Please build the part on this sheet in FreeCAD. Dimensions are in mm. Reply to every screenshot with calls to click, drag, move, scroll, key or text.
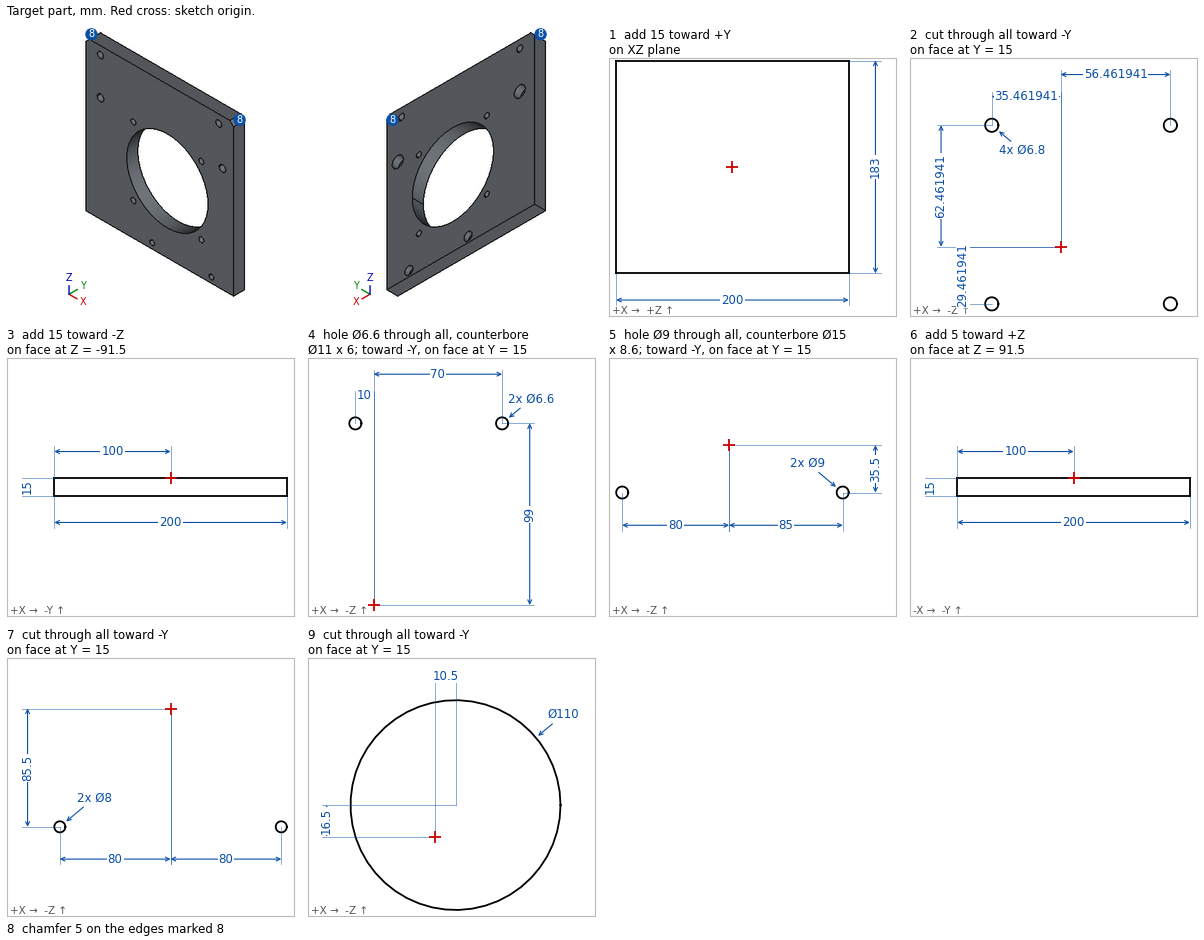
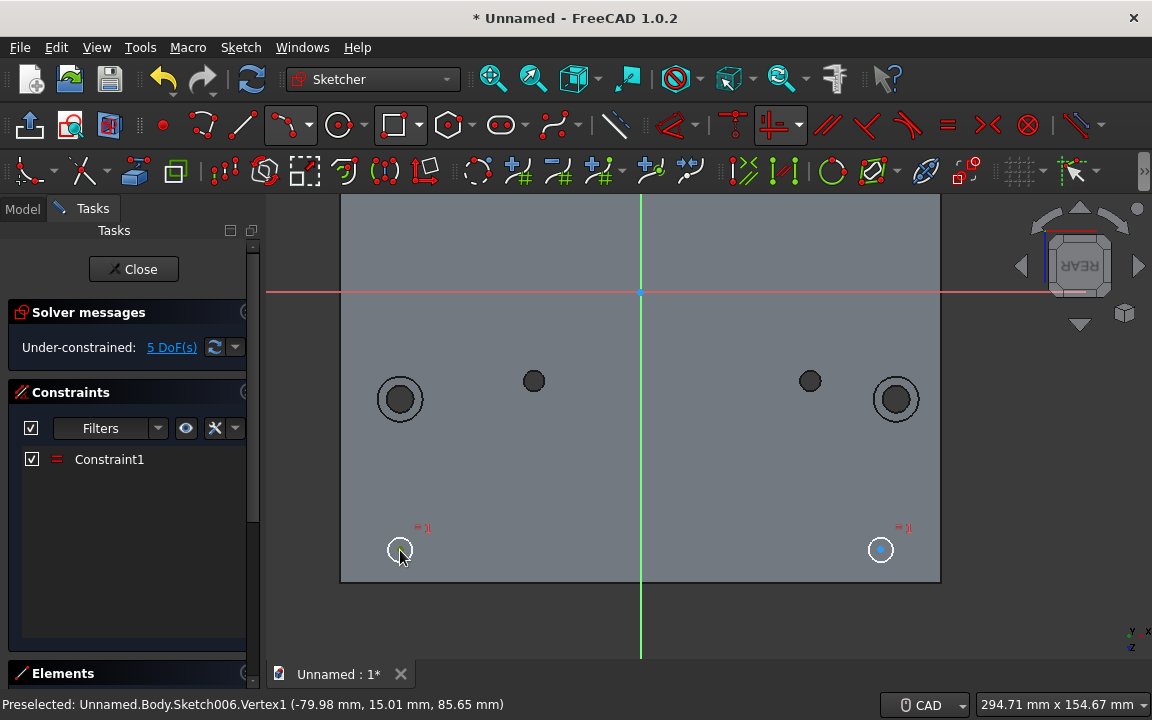
click(881, 550)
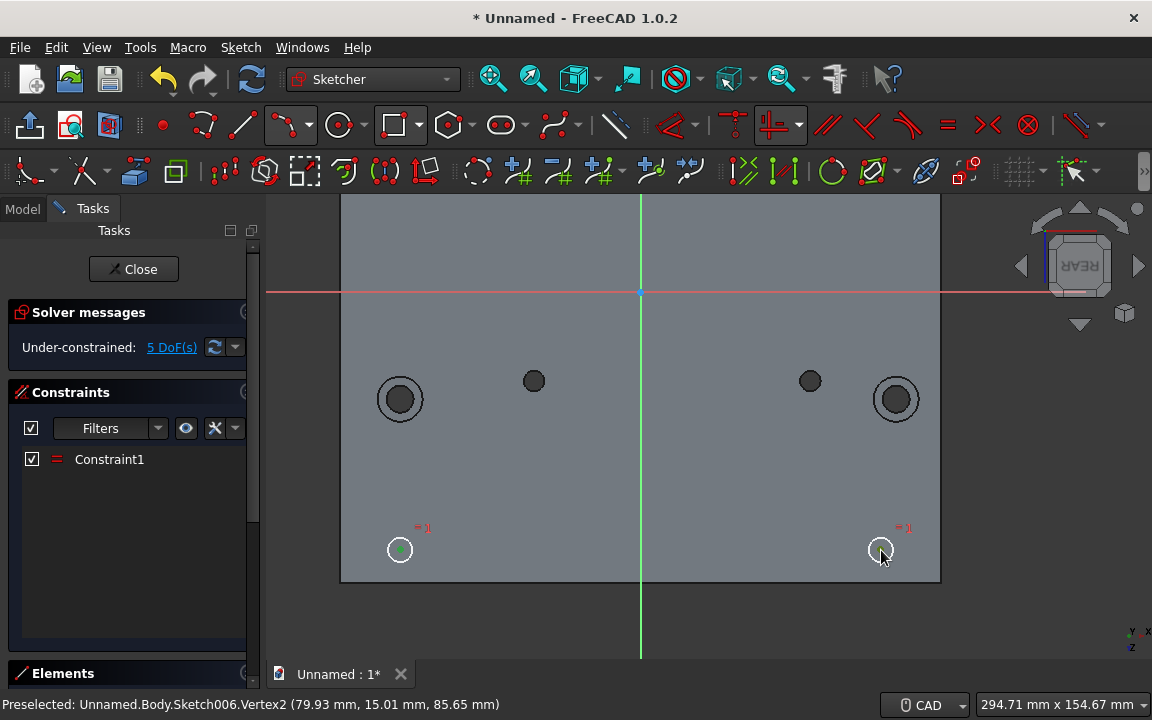
key(h)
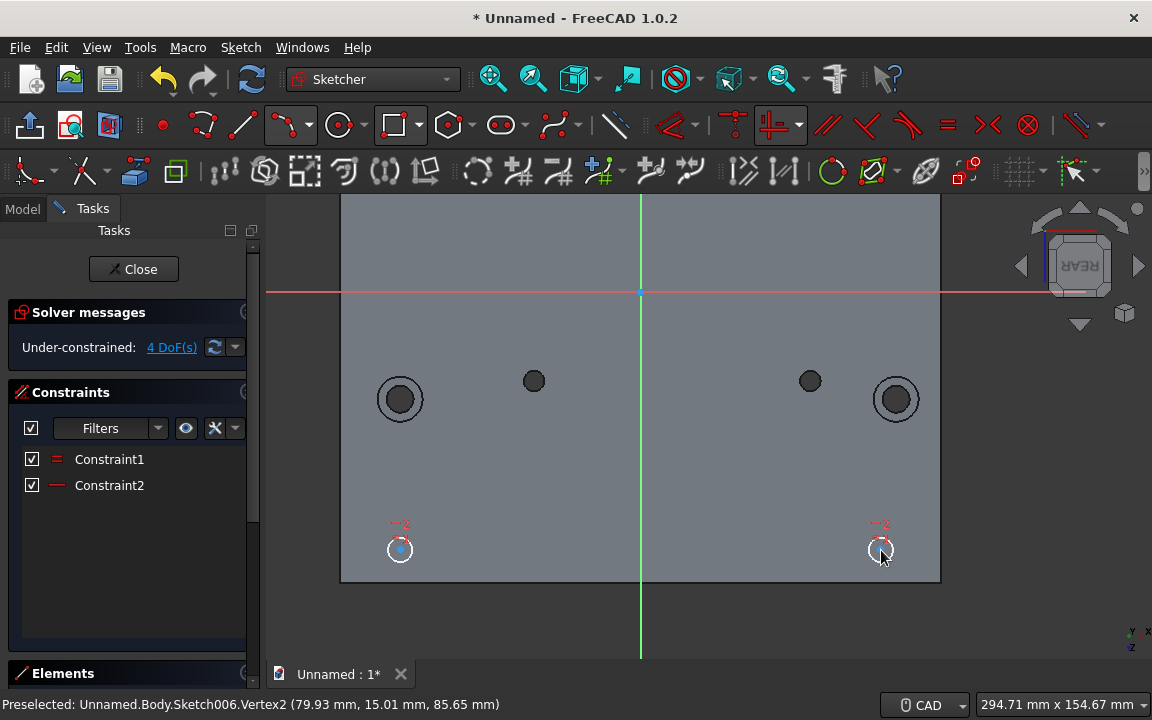
click(670, 126)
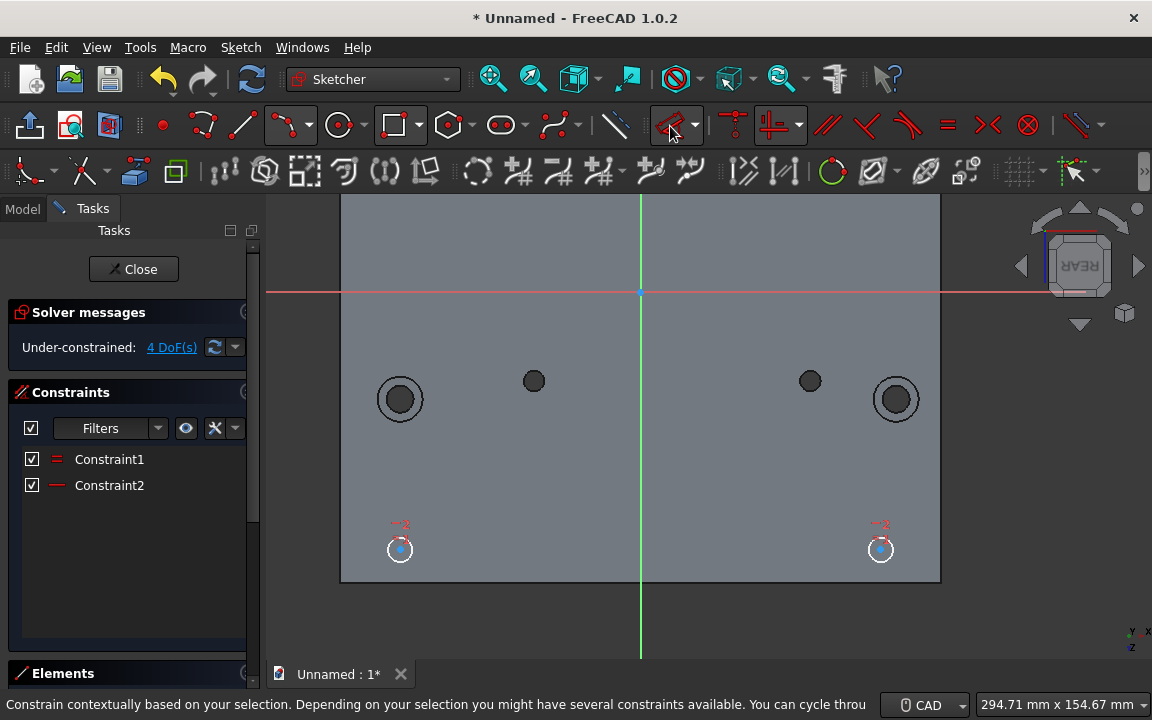
scroll(409, 541, up, 3)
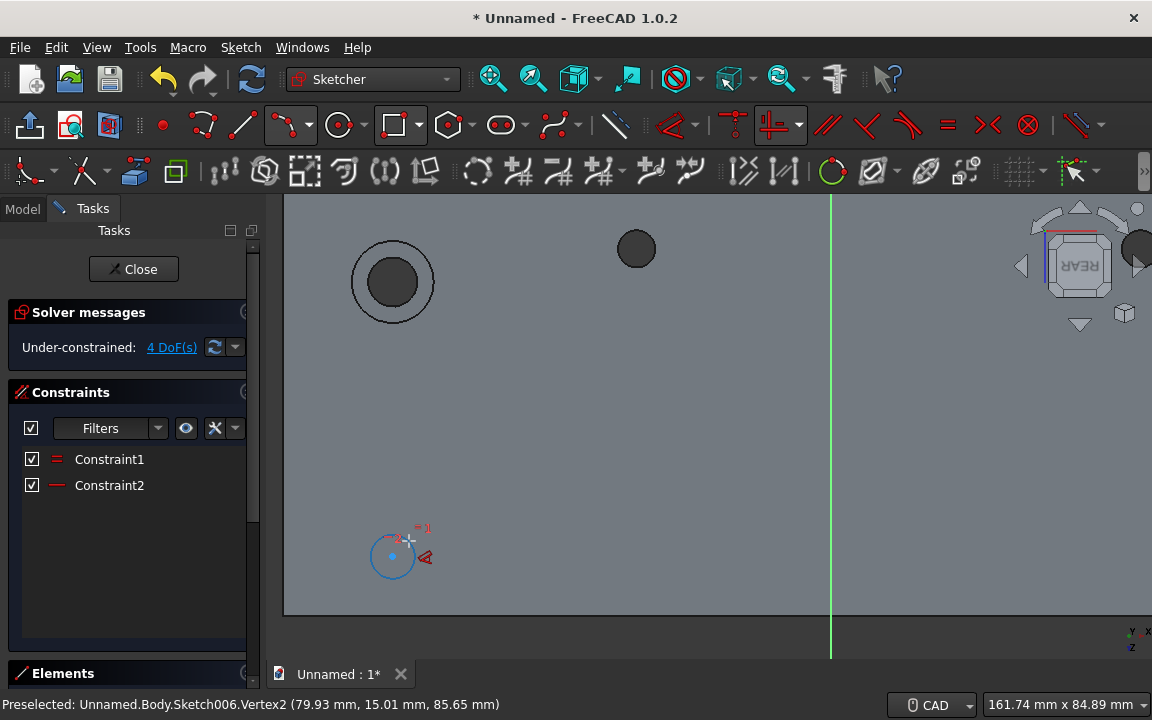
click(408, 541)
click(430, 518)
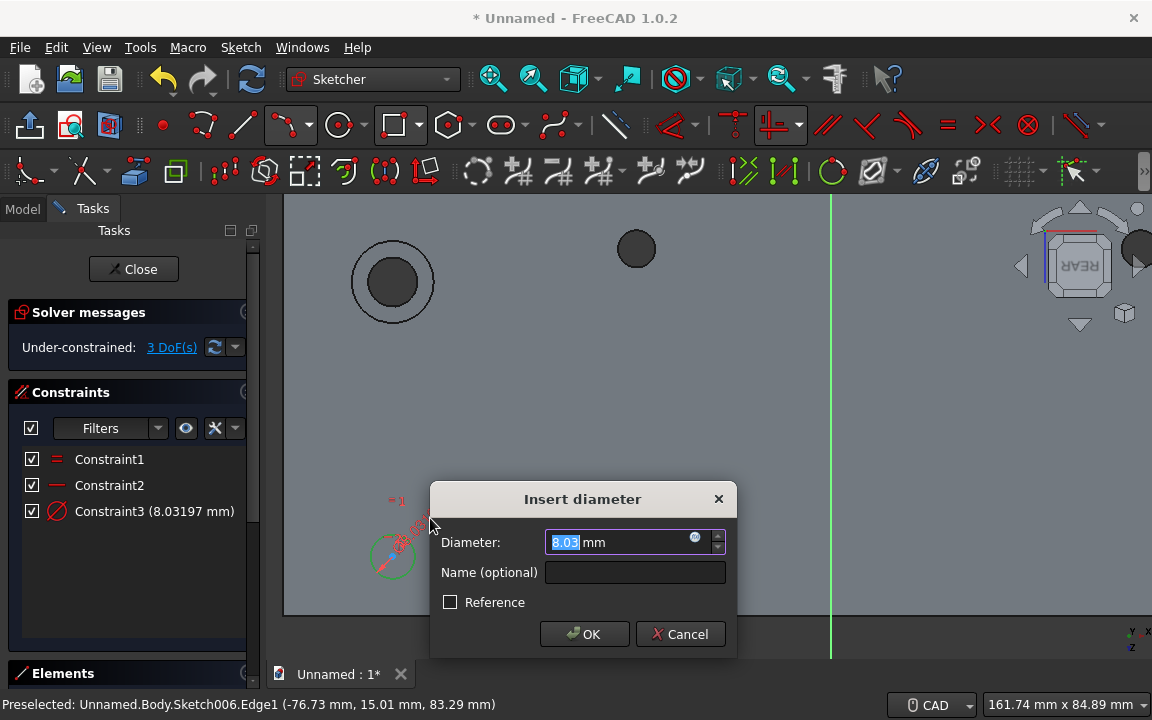
text(8)
key(Return)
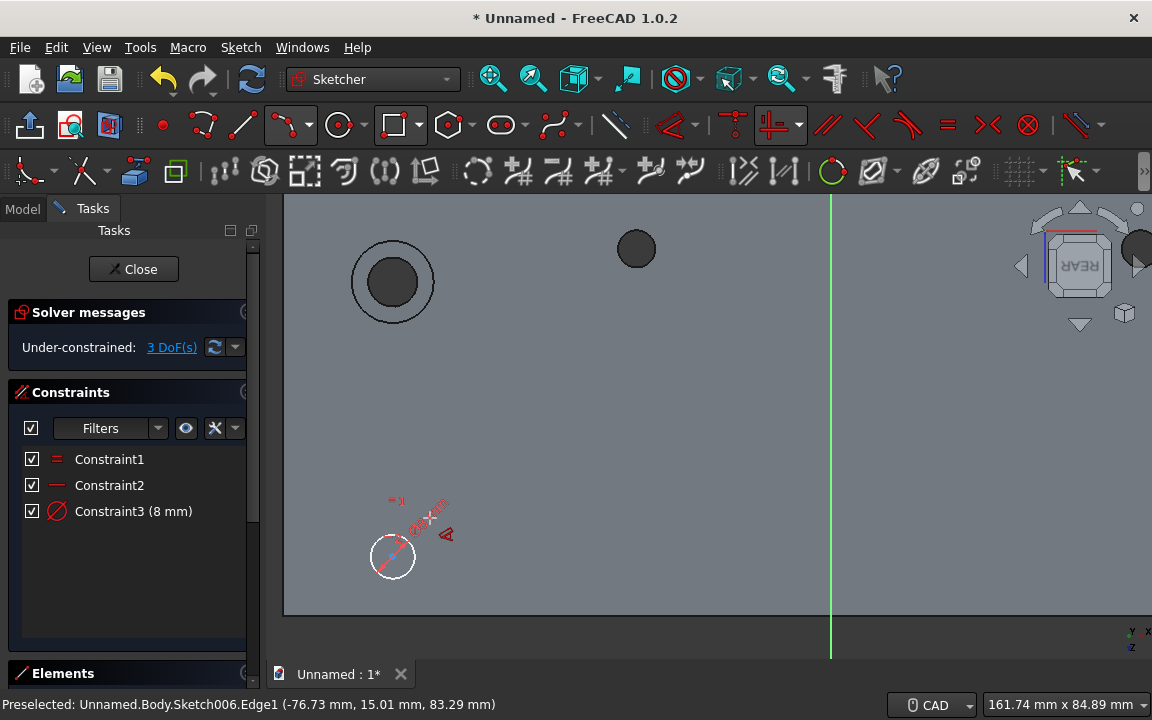
click(393, 557)
click(612, 591)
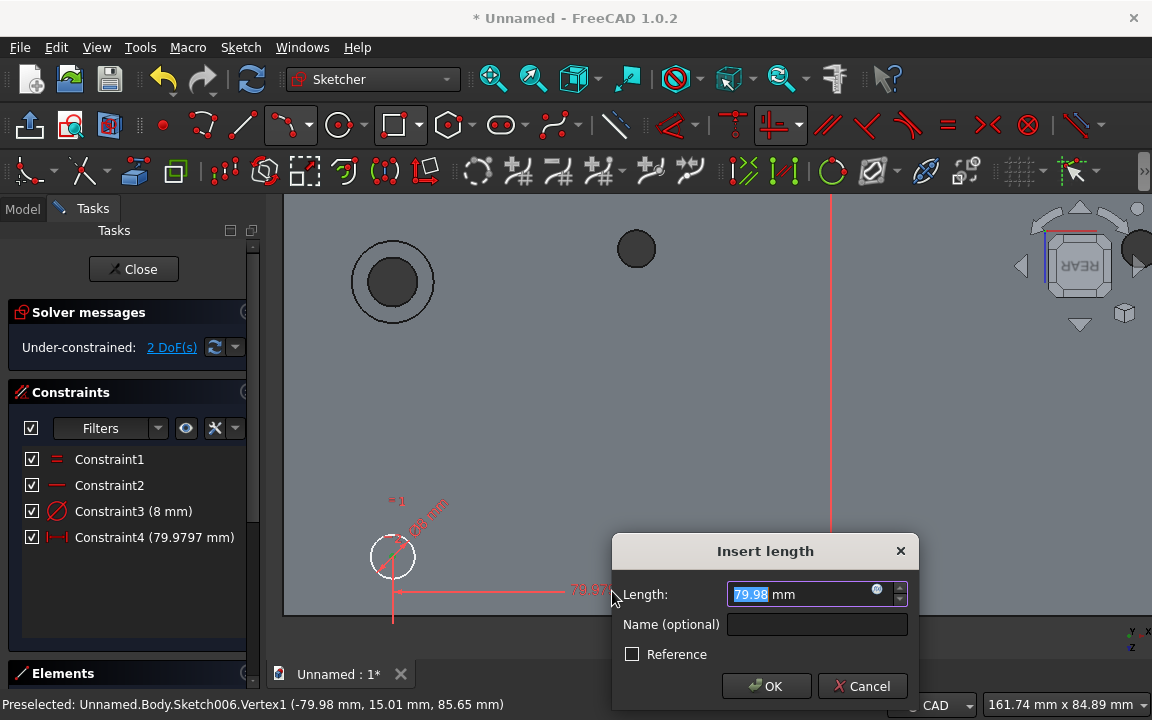
text(80)
key(Return)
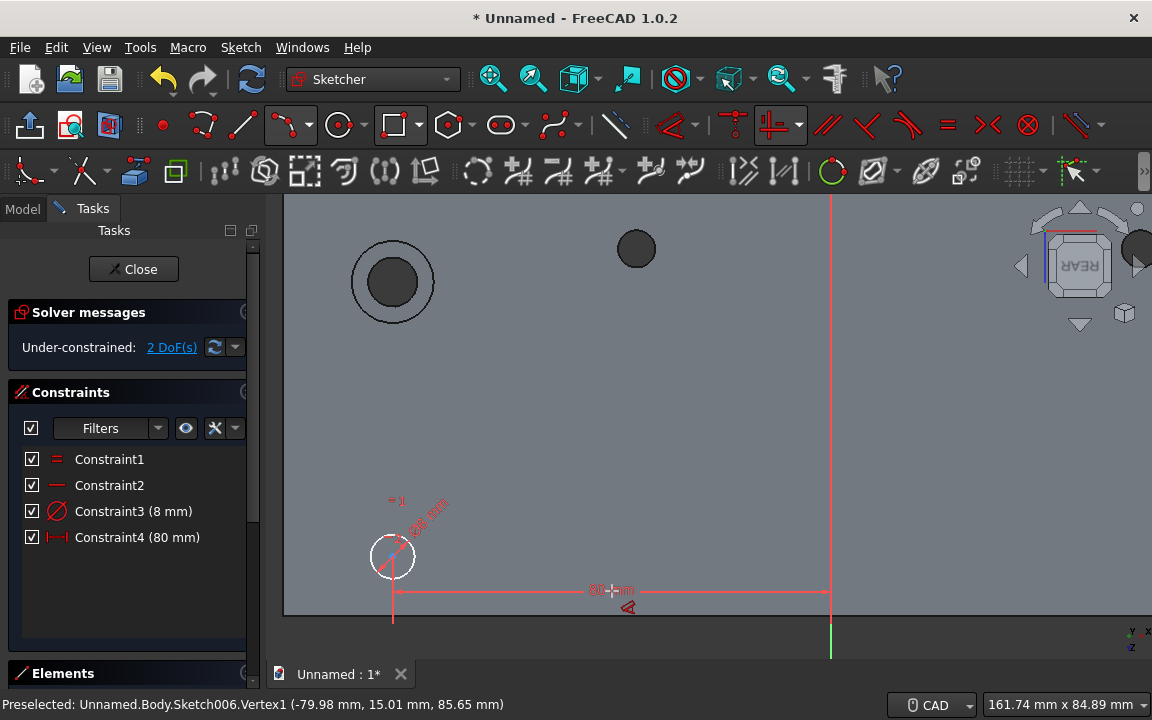
scroll(409, 541, down, 3)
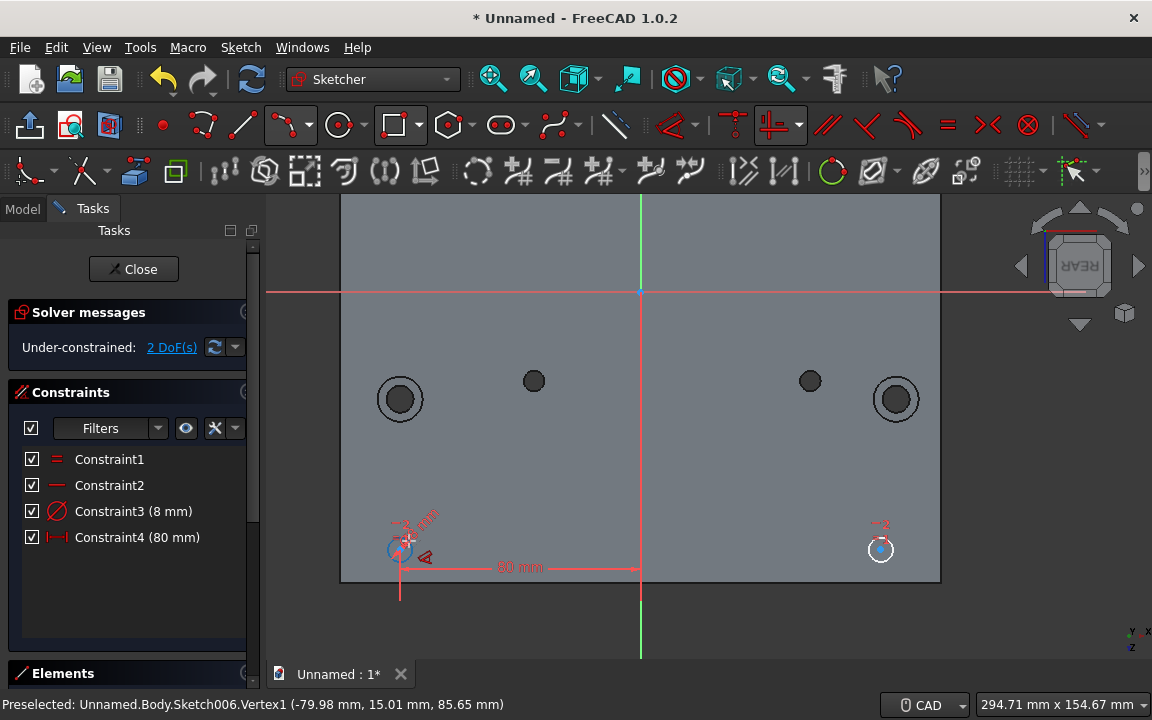
click(881, 550)
click(761, 258)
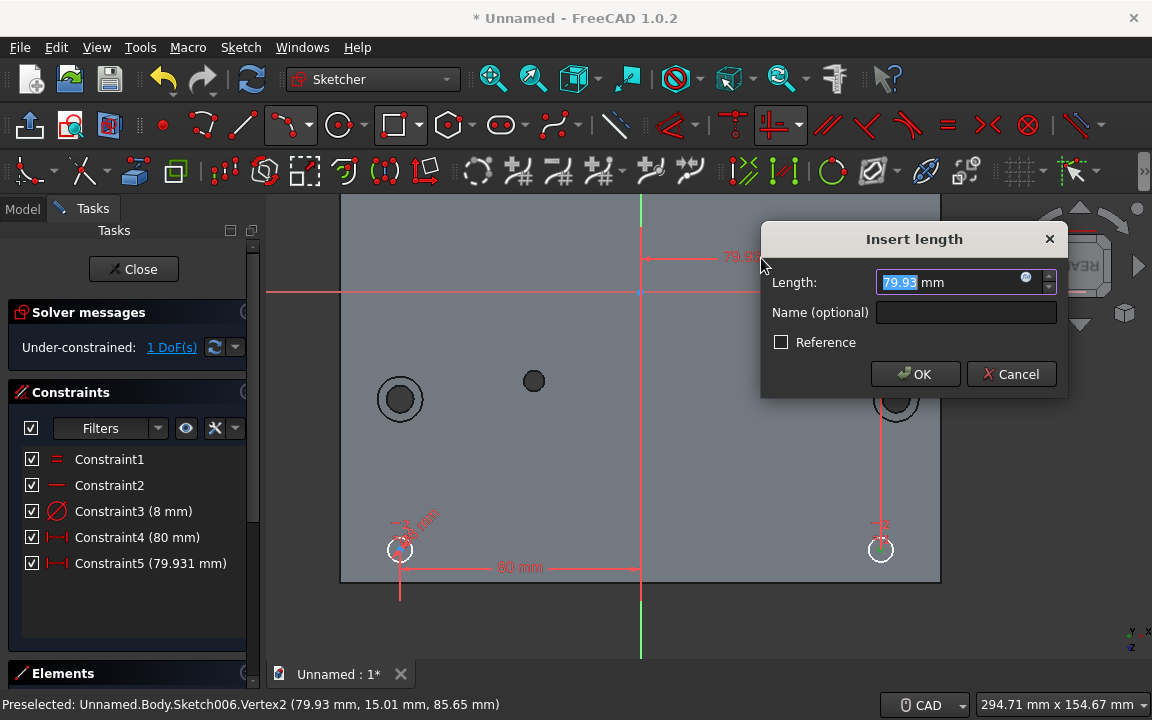
text(80)
key(Return)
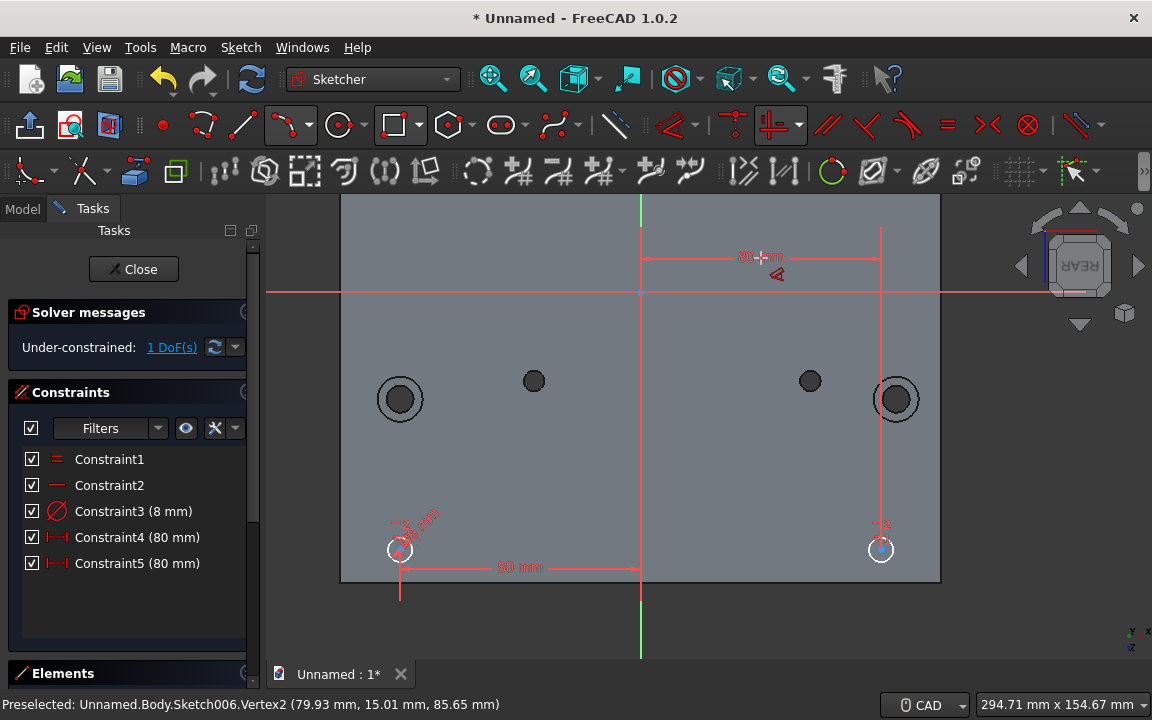
click(400, 550)
click(366, 421)